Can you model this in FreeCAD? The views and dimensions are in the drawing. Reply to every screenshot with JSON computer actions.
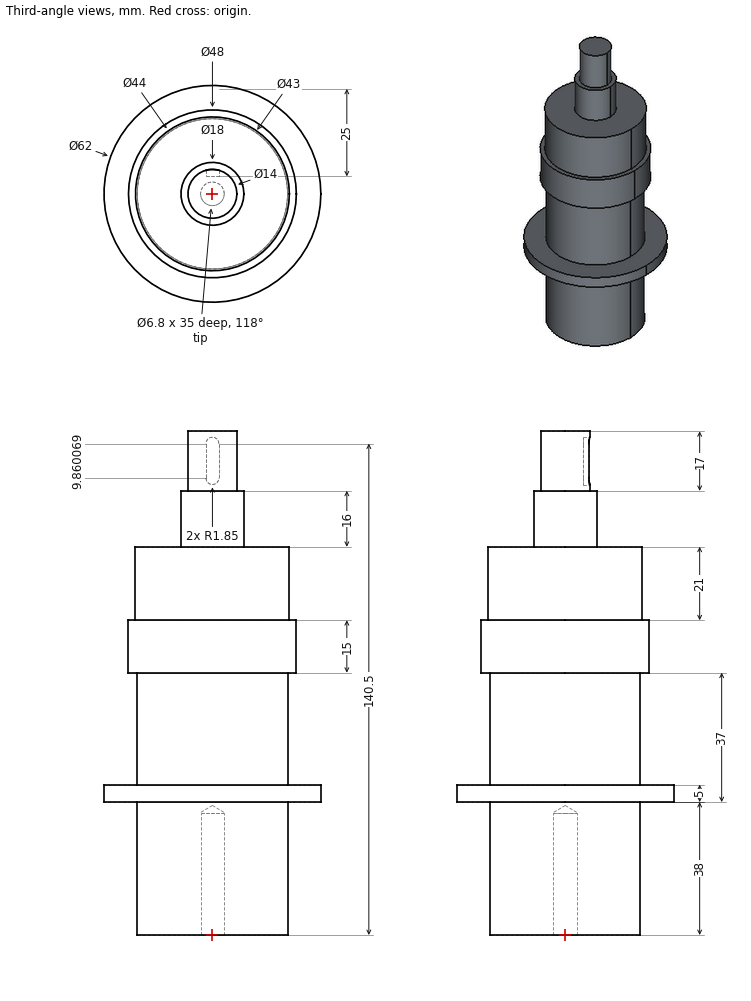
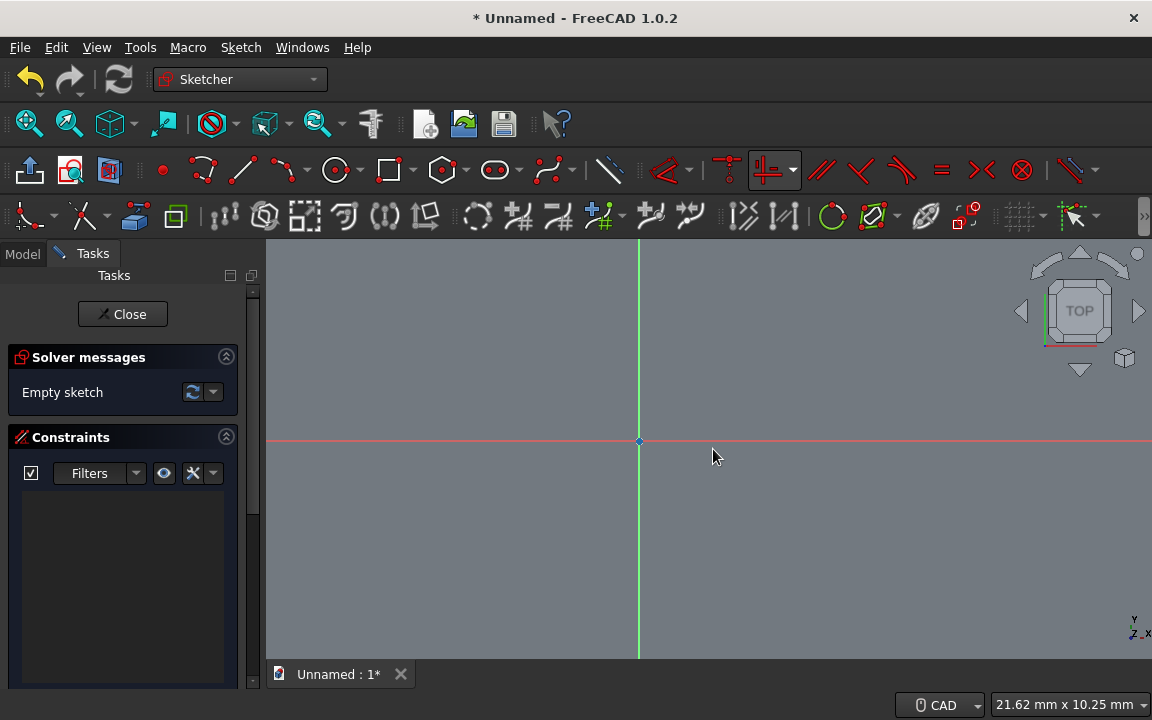
{"action": "left_click", "coordinate": [336, 170]}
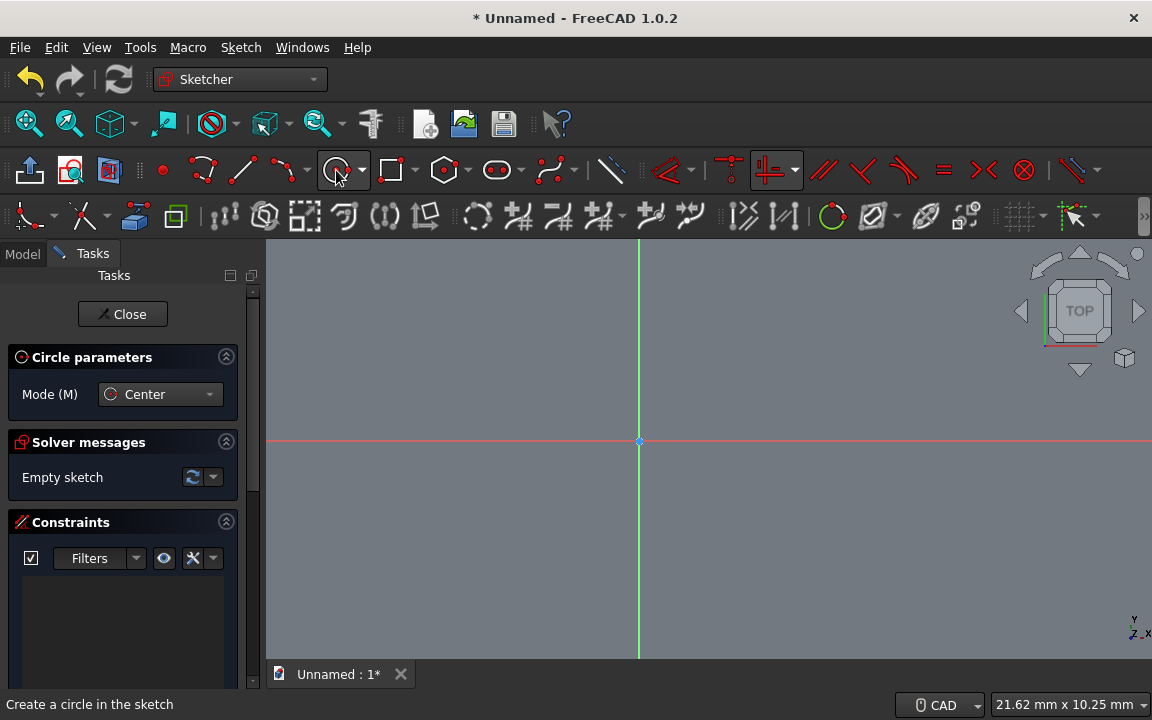
{"action": "left_click", "coordinate": [639, 441]}
{"action": "left_click", "coordinate": [738, 343]}
{"action": "key", "text": "Escape"}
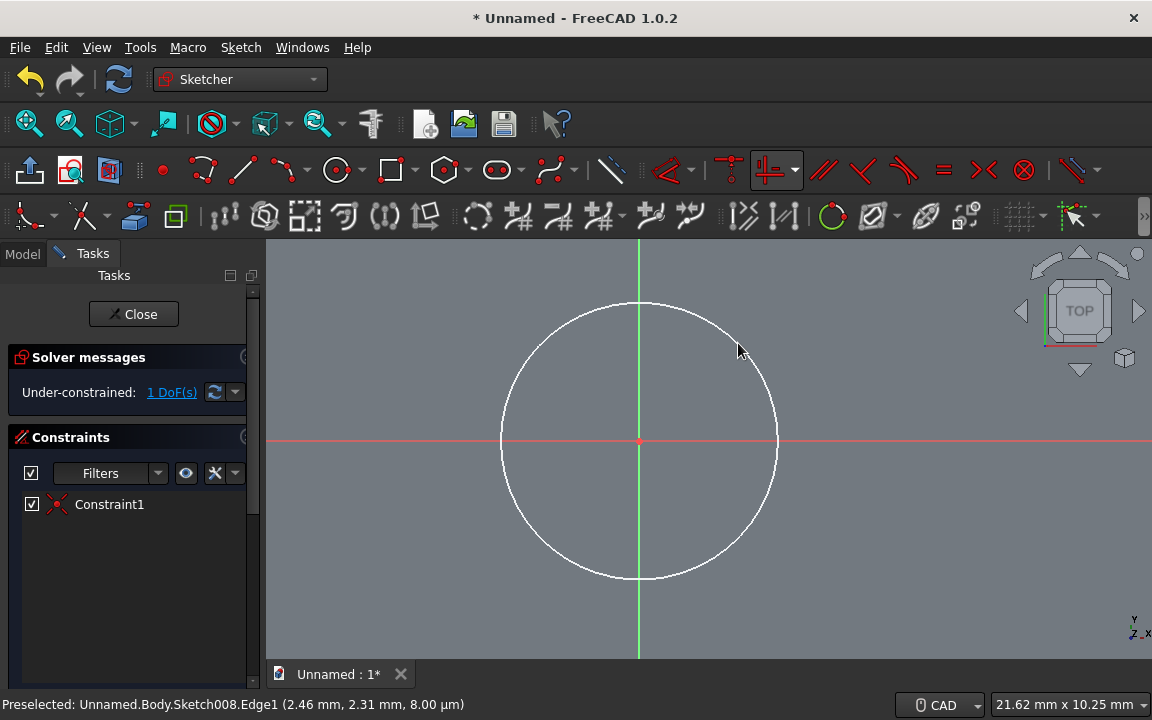
{"action": "key", "text": "d"}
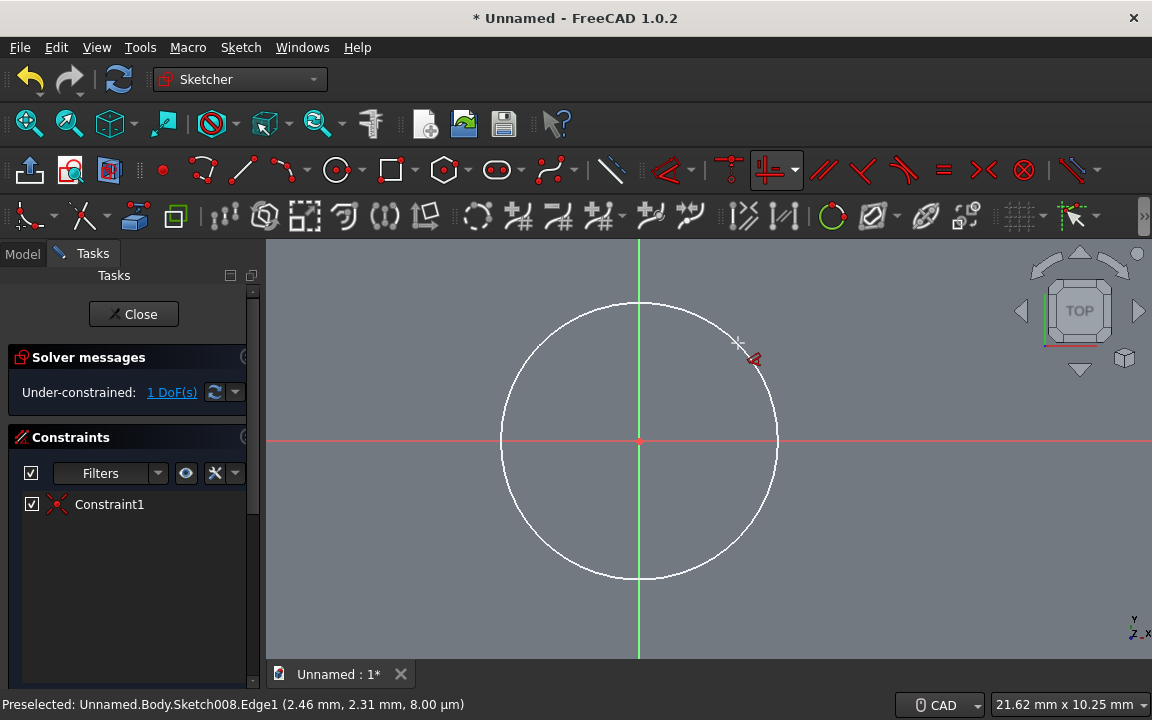
{"action": "left_click", "coordinate": [737, 343]}
{"action": "left_click", "coordinate": [760, 320]}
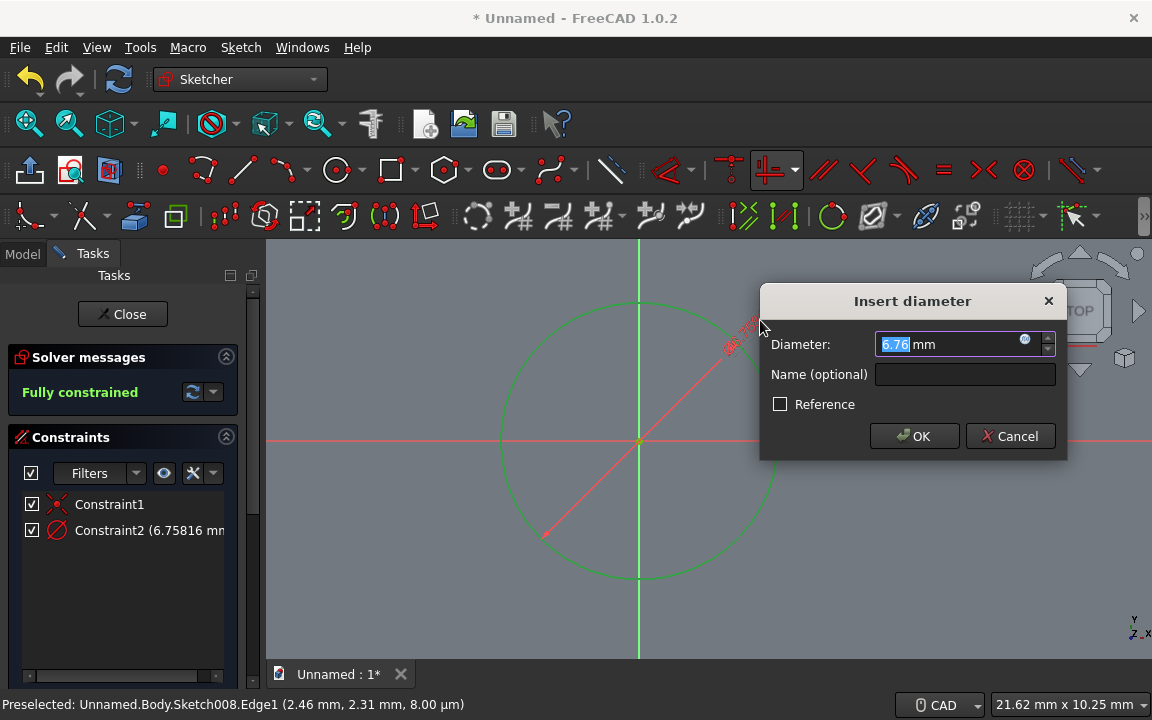
{"action": "type", "text": "6.8"}
{"action": "key", "text": "Return"}
{"action": "key", "text": "Escape"}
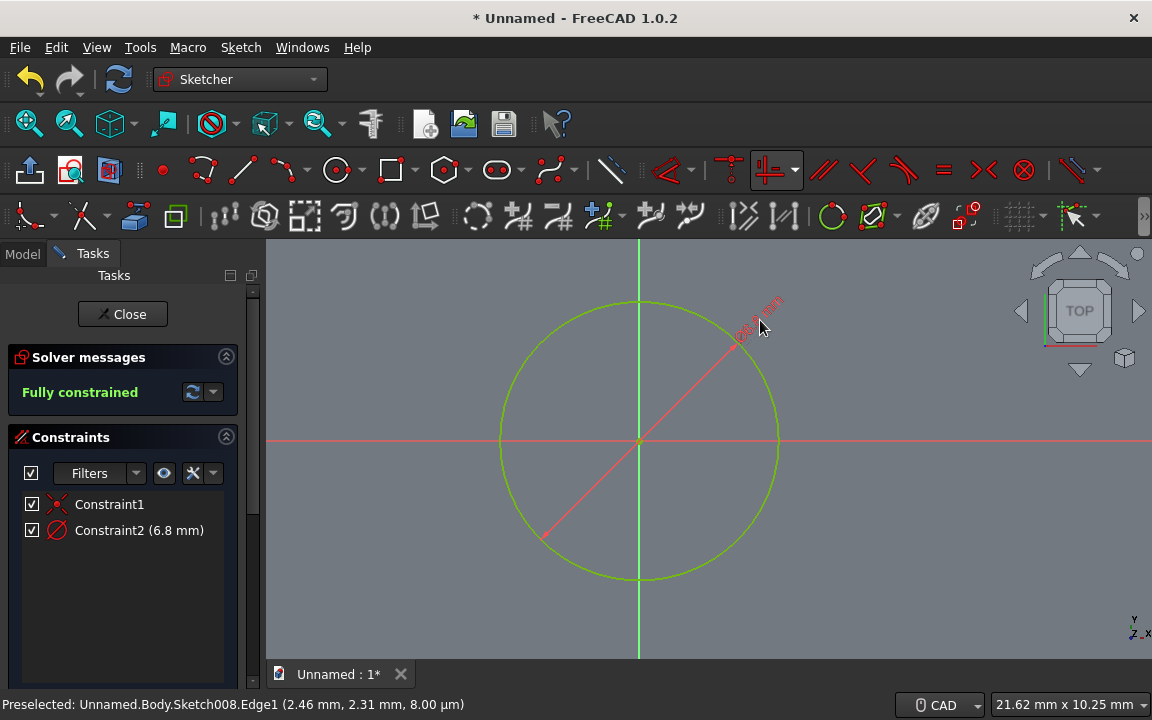
{"action": "left_click", "coordinate": [123, 314]}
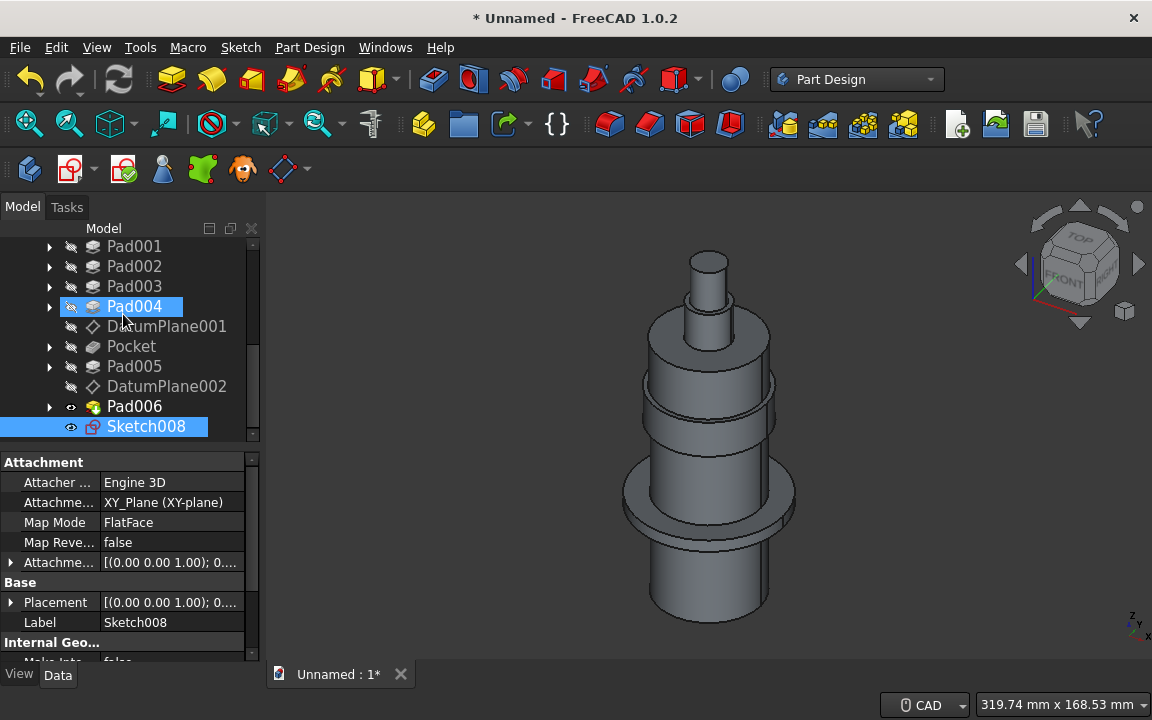
{"action": "left_click", "coordinate": [474, 80]}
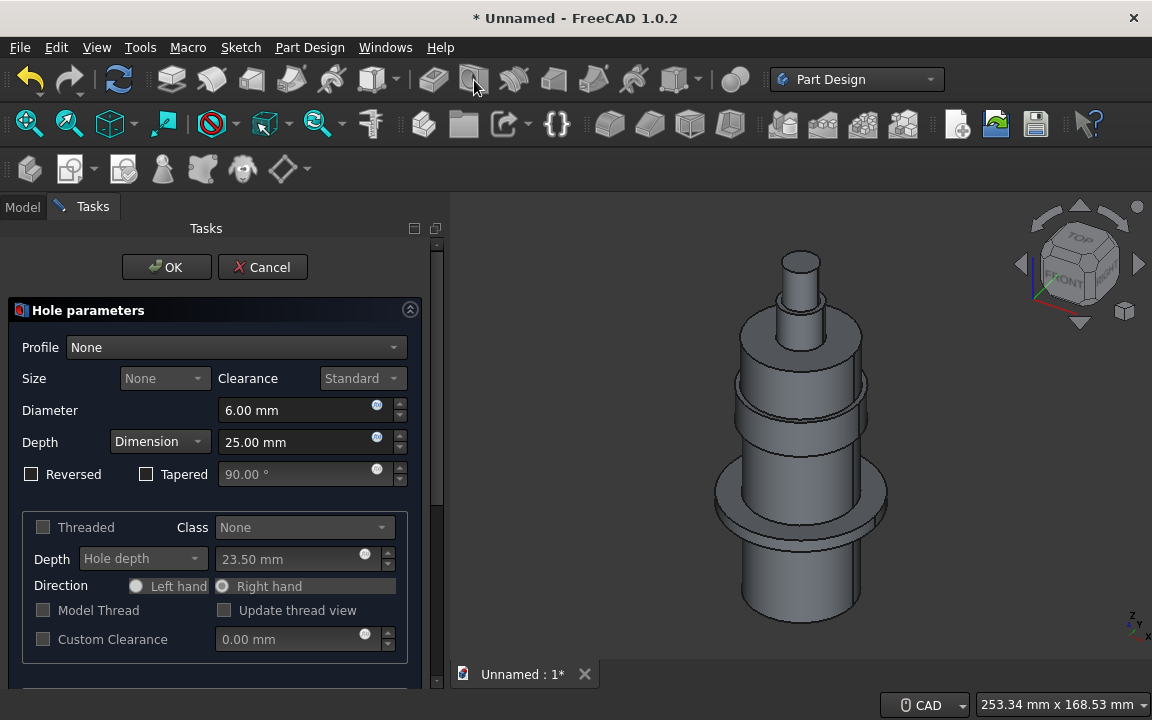
{"action": "triple_click", "coordinate": [305, 410]}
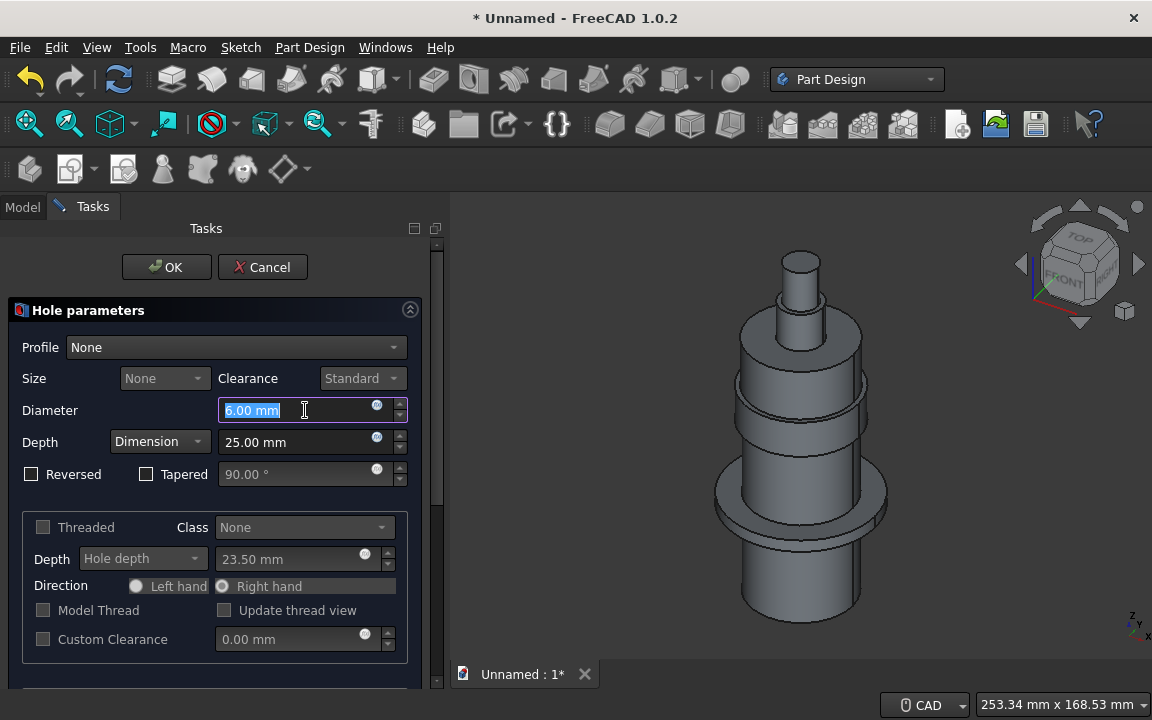
{"action": "type", "text": "6.8"}
{"action": "key", "text": "Tab"}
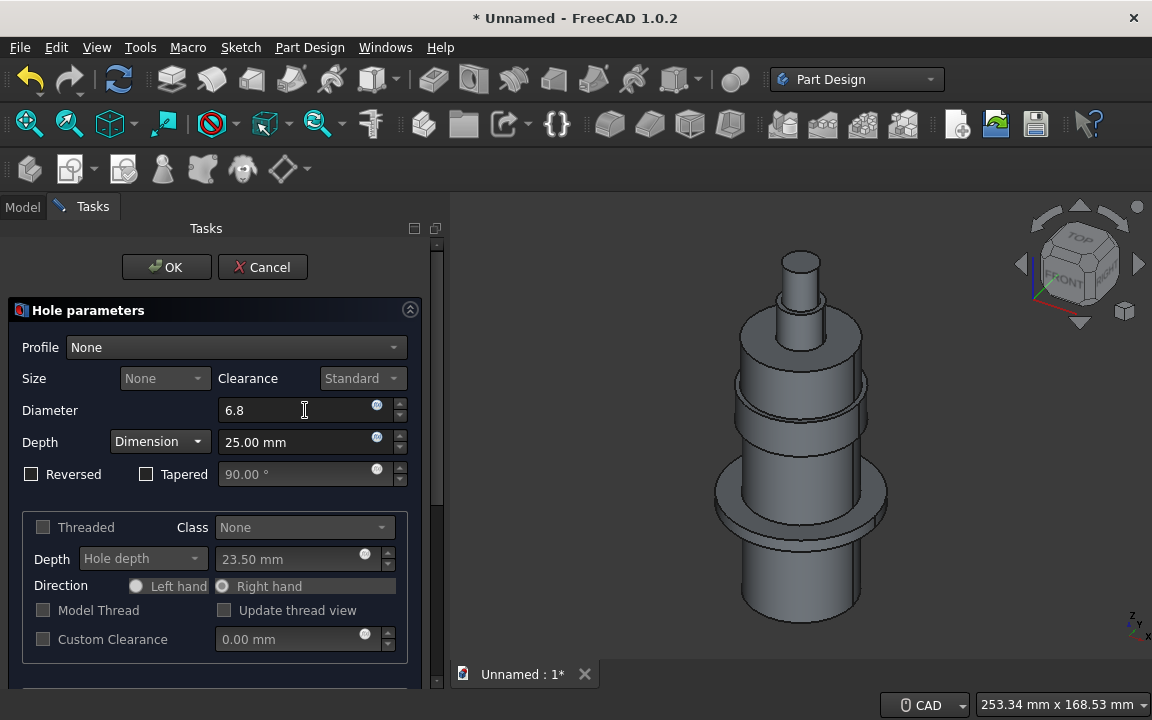
{"action": "triple_click", "coordinate": [305, 442]}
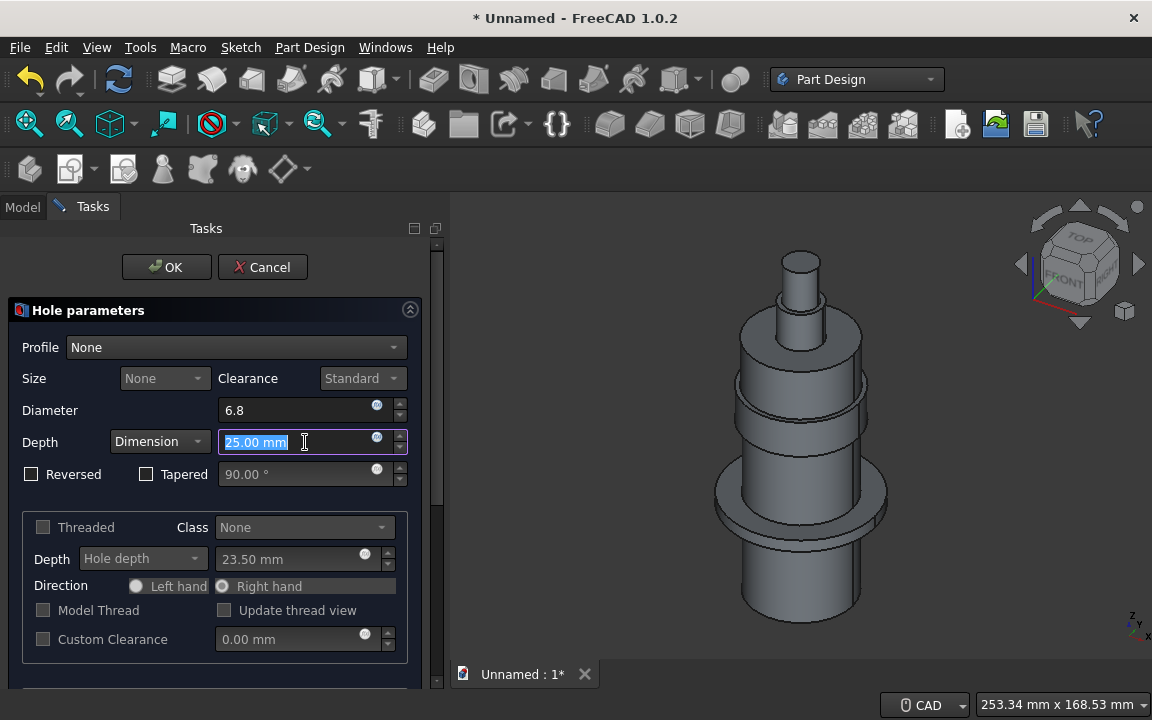
{"action": "type", "text": "35"}
{"action": "key", "text": "Tab"}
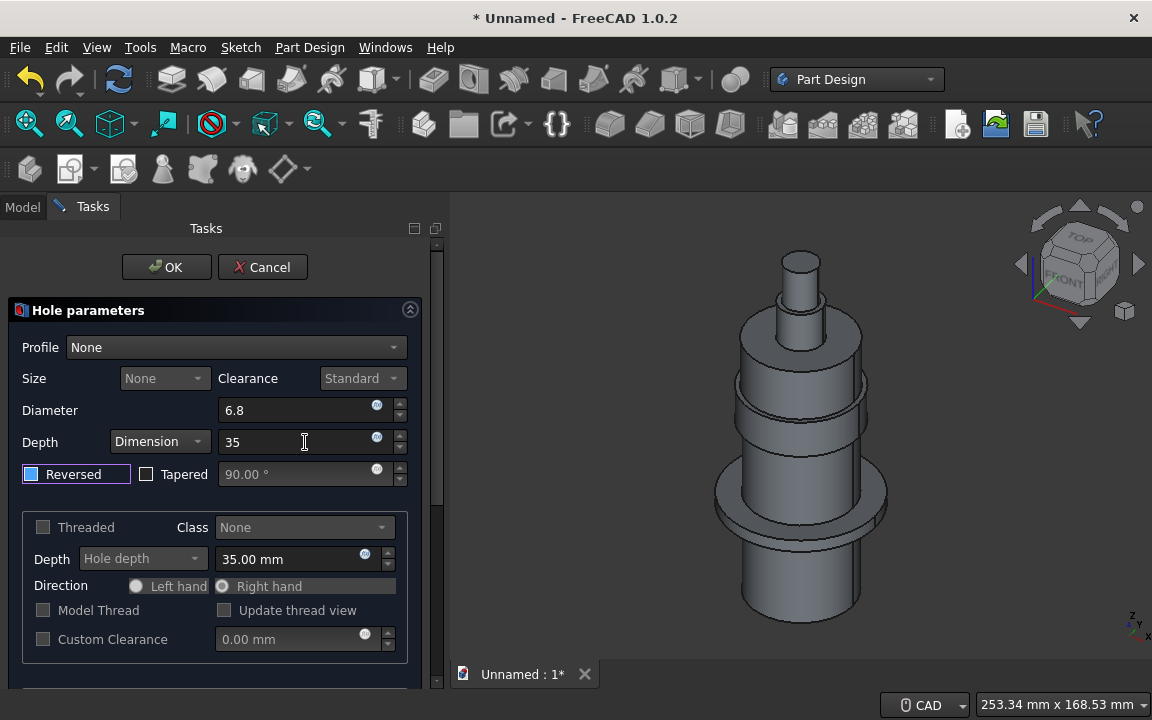
{"action": "left_click", "coordinate": [30, 474]}